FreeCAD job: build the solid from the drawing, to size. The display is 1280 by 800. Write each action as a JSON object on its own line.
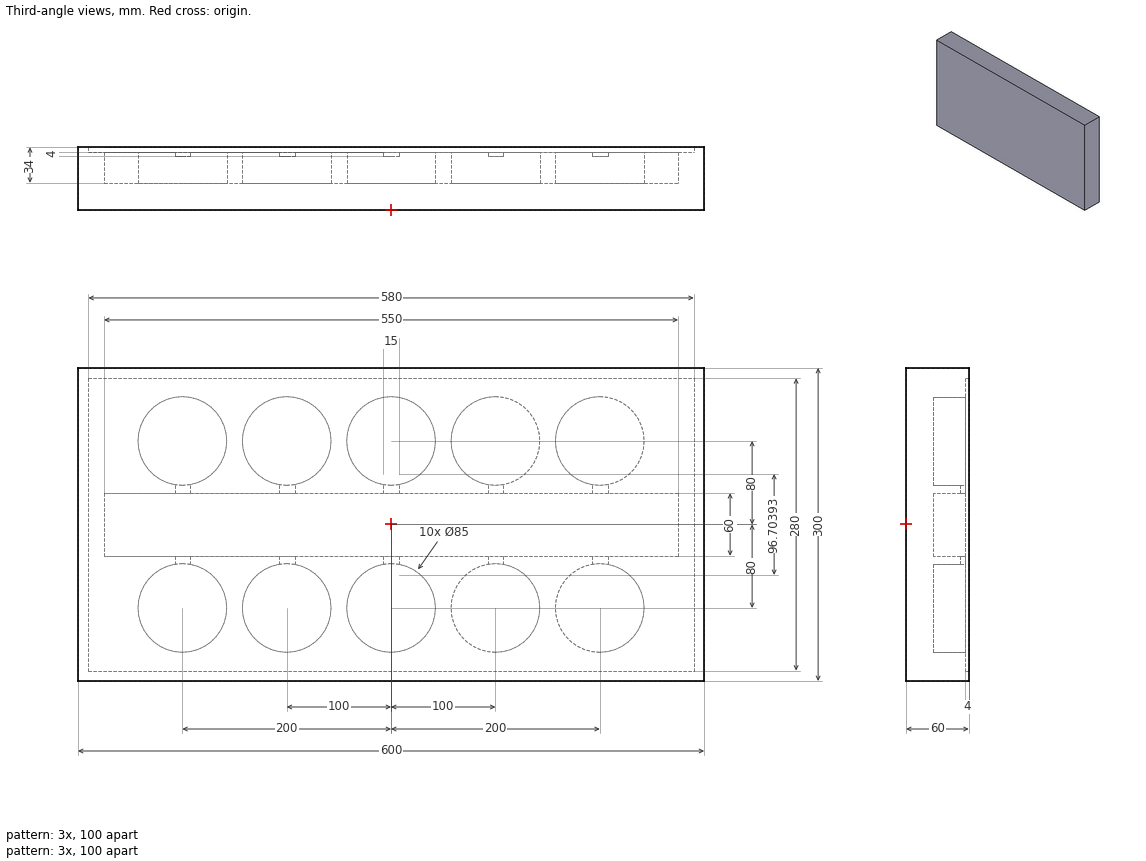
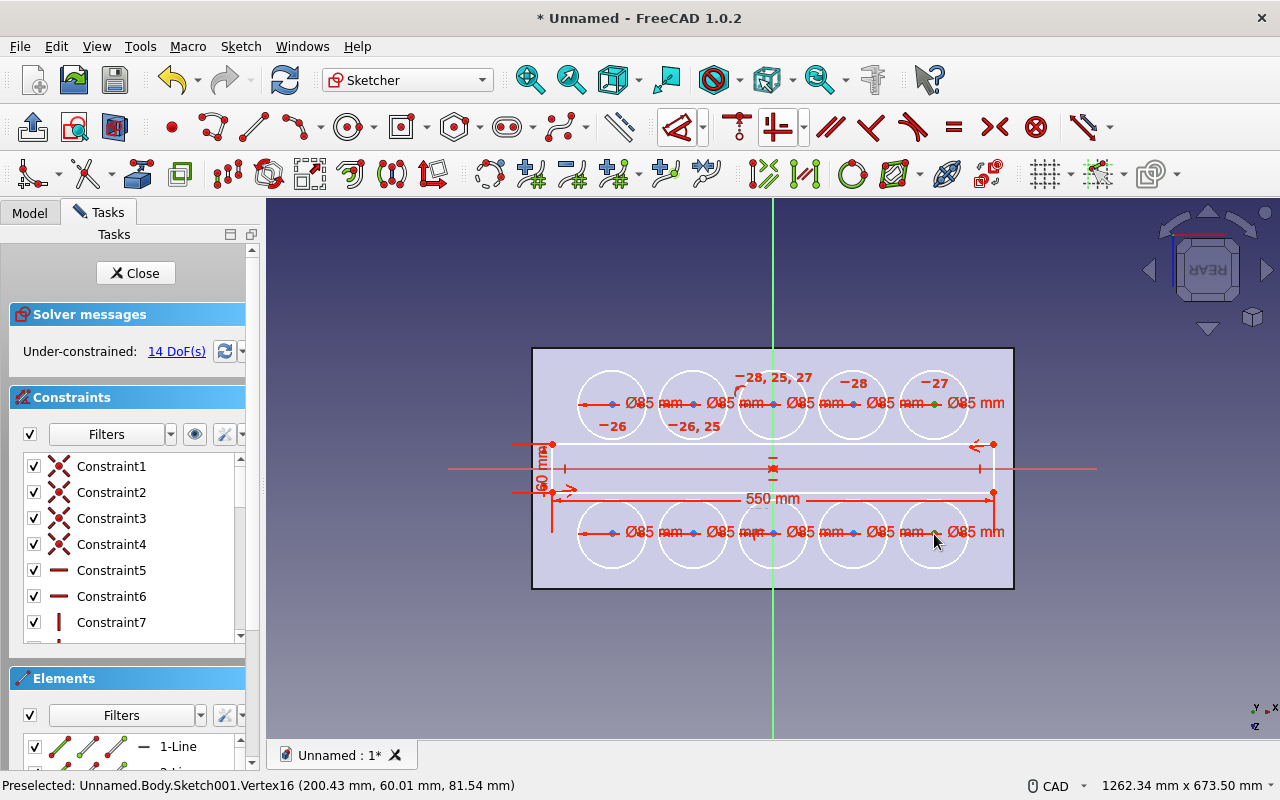
{"action": "left_click", "coordinate": [804, 128]}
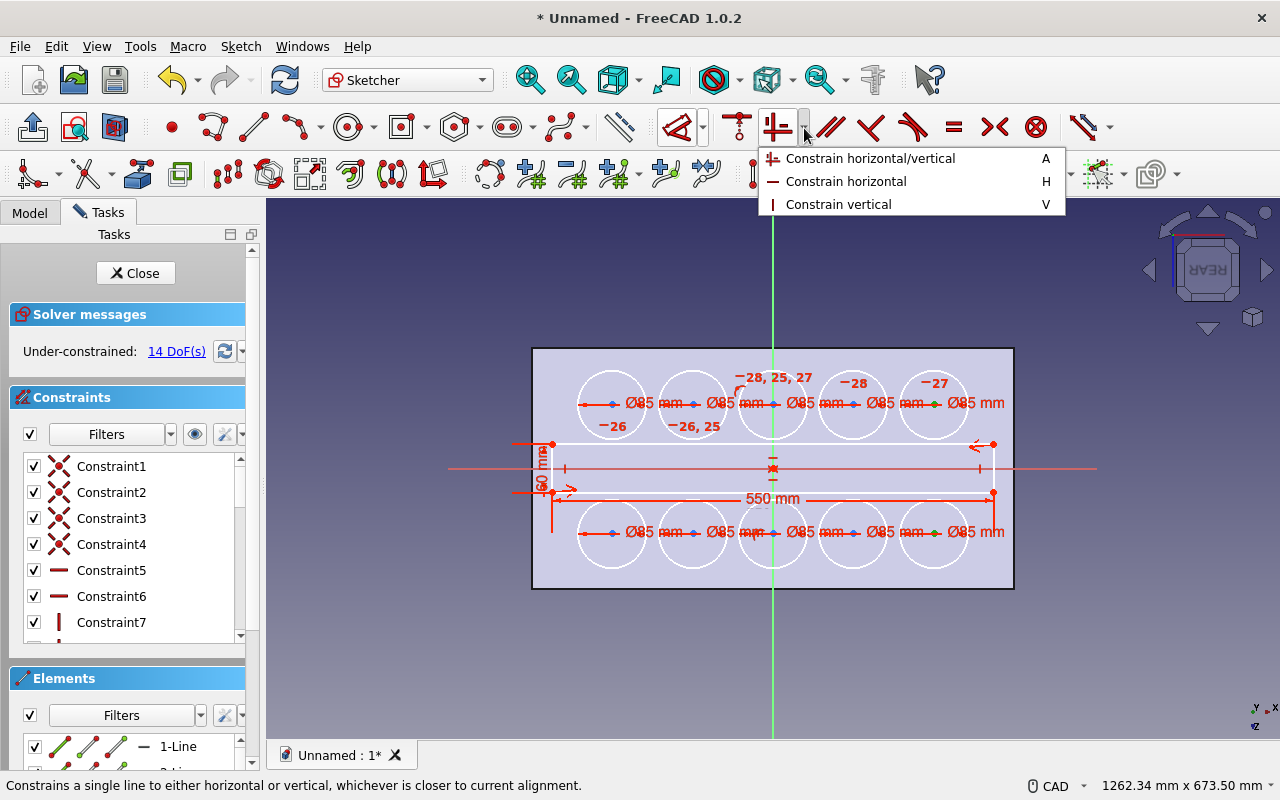
{"action": "left_click", "coordinate": [912, 204]}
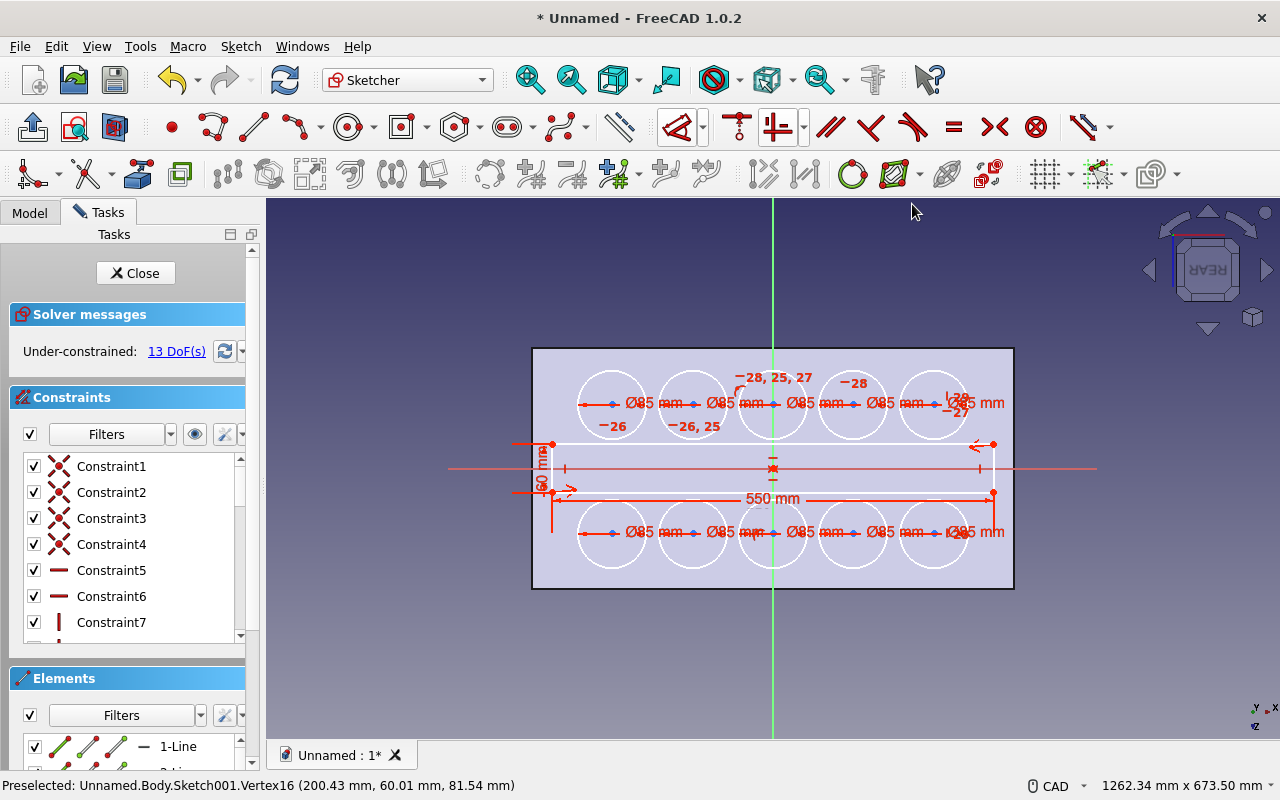
{"action": "left_click", "coordinate": [853, 405]}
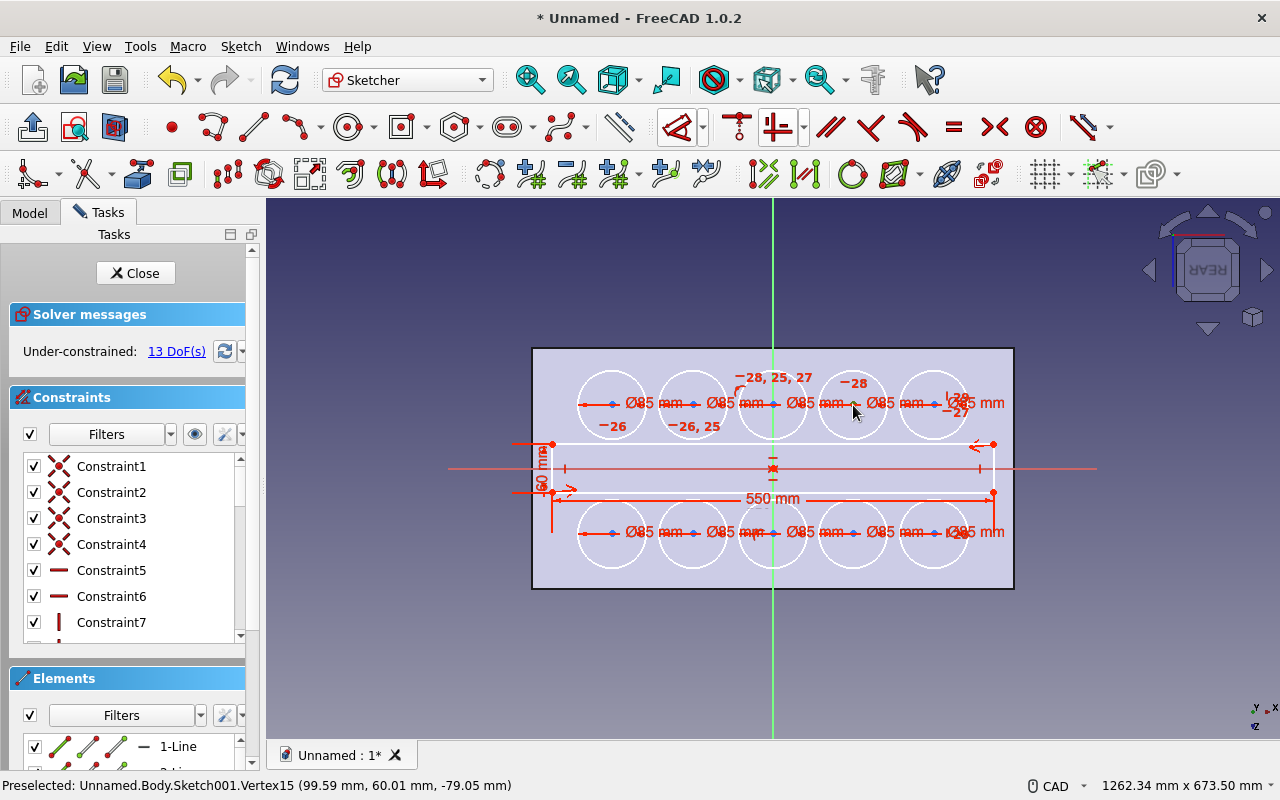
{"action": "left_click", "coordinate": [853, 534]}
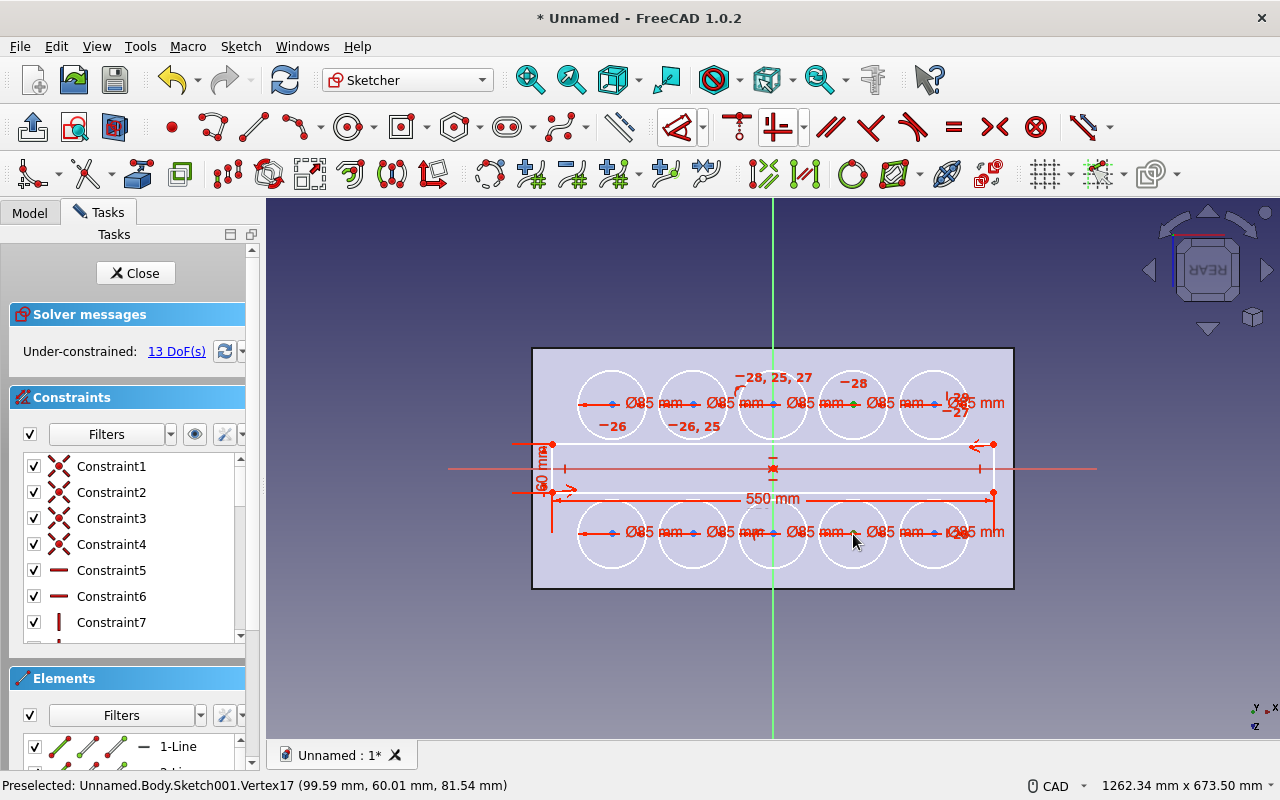
{"action": "key", "text": "v"}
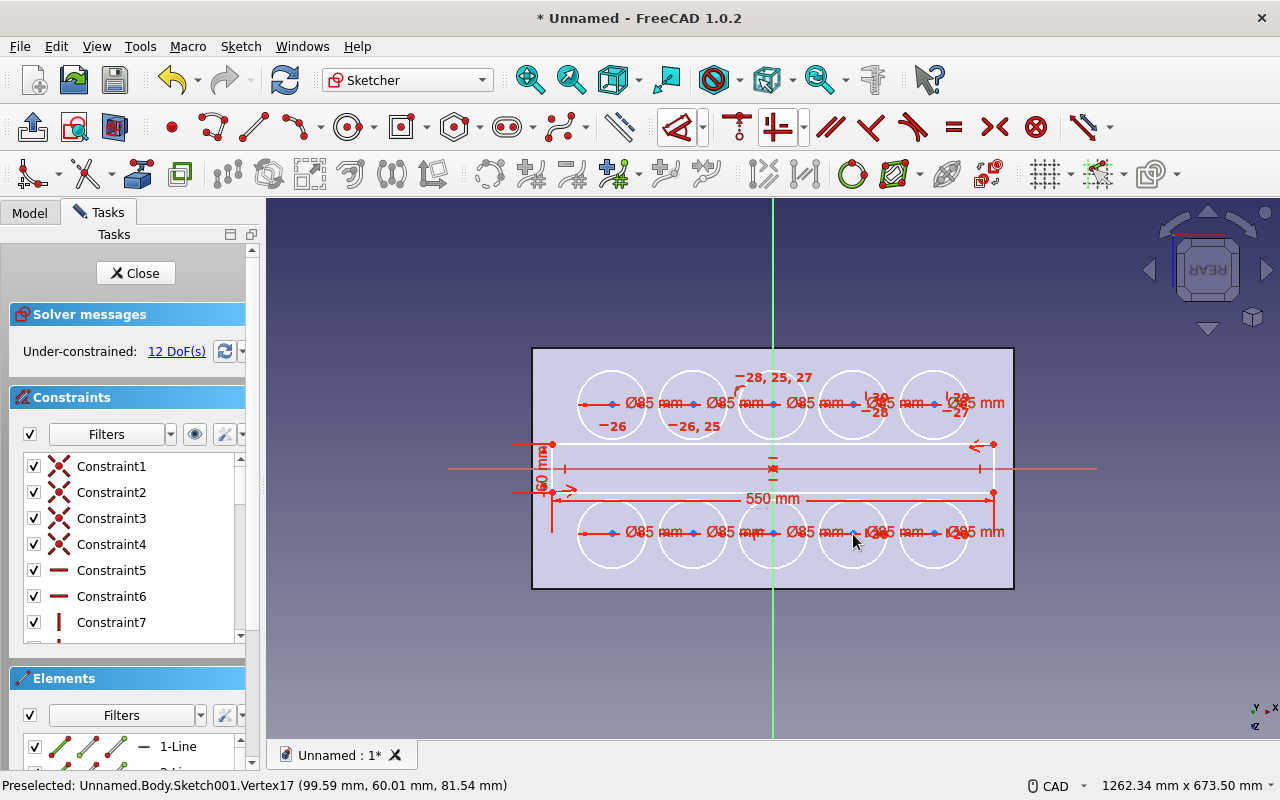
{"action": "left_click", "coordinate": [773, 534]}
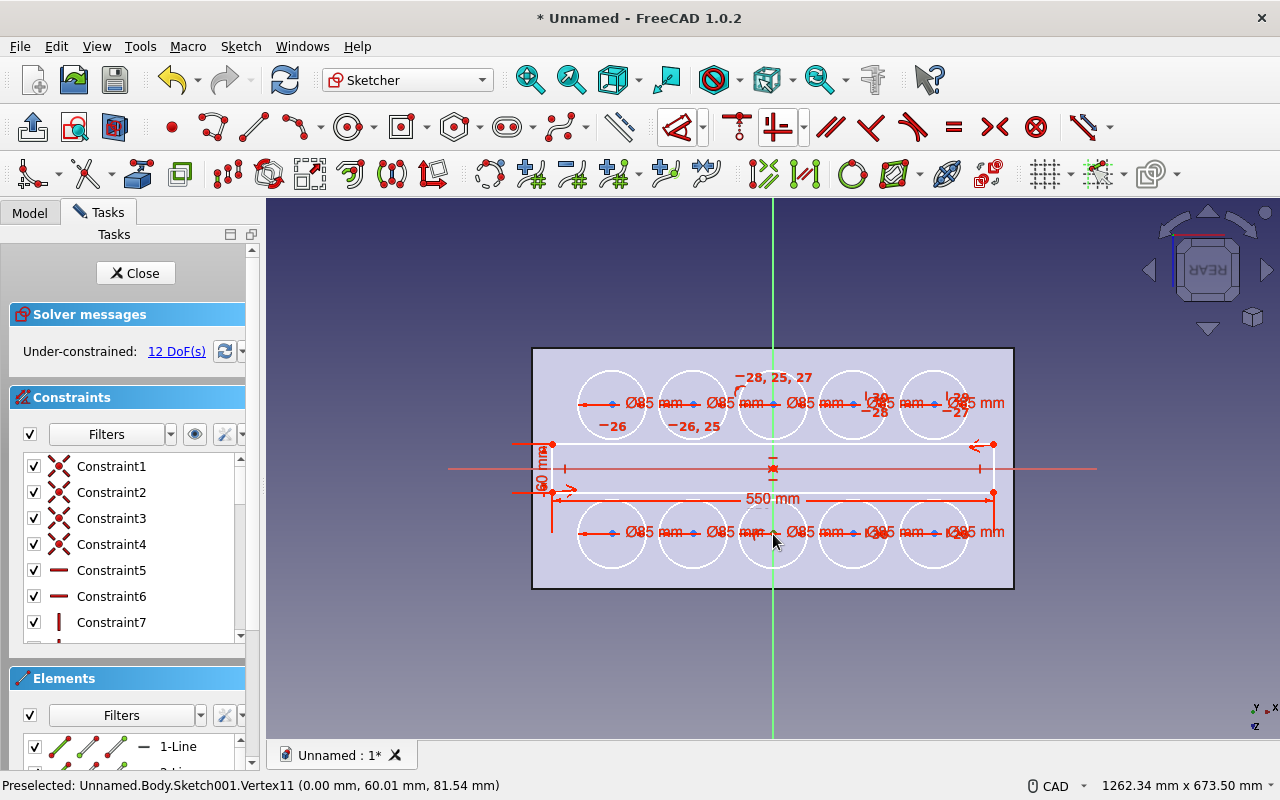
{"action": "left_click", "coordinate": [853, 534]}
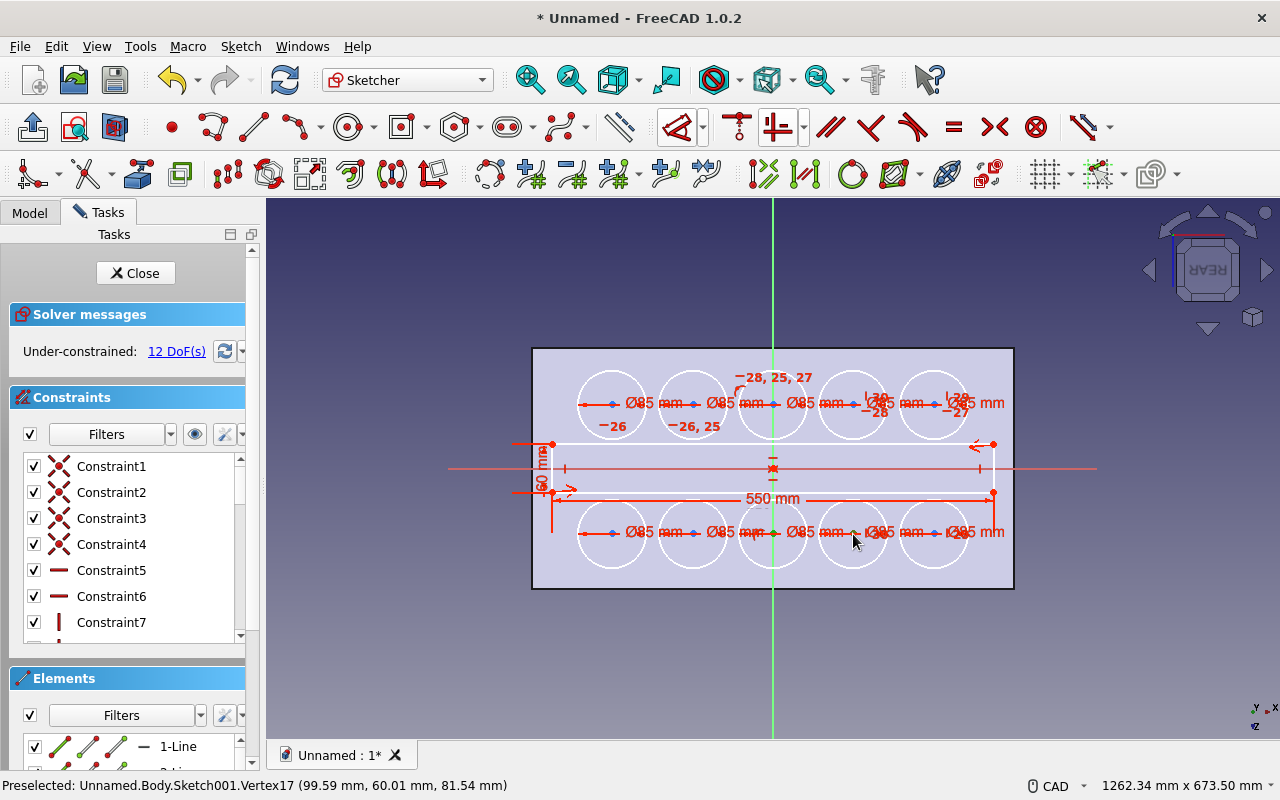
{"action": "key", "text": "h"}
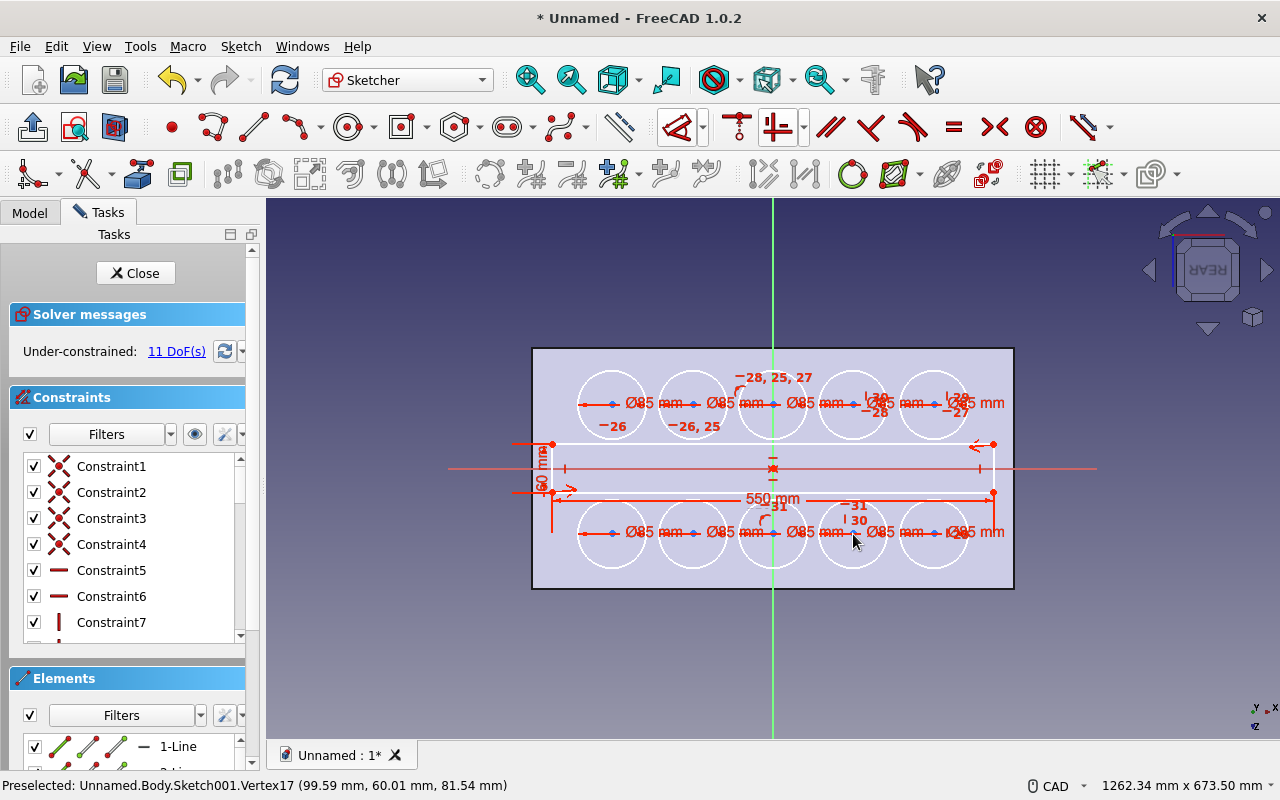
{"action": "left_click", "coordinate": [934, 534]}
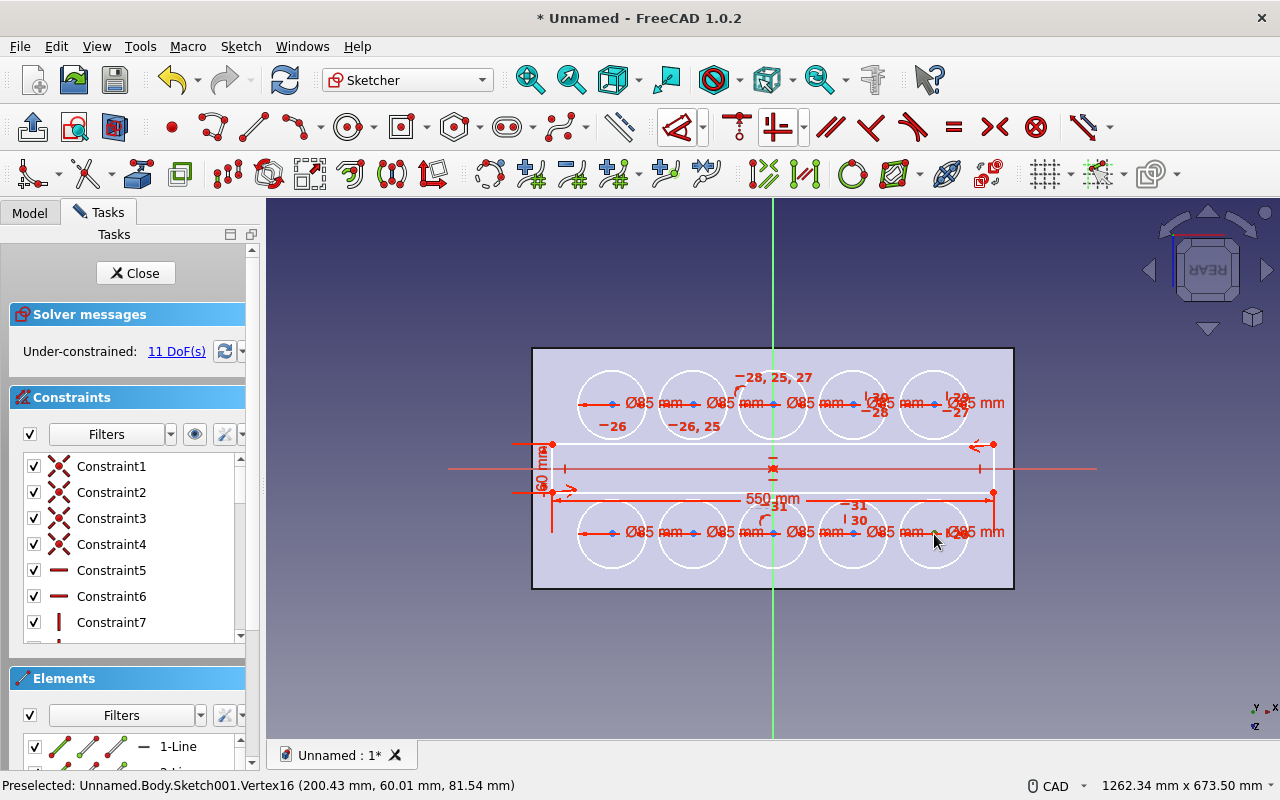
{"action": "left_click", "coordinate": [853, 534]}